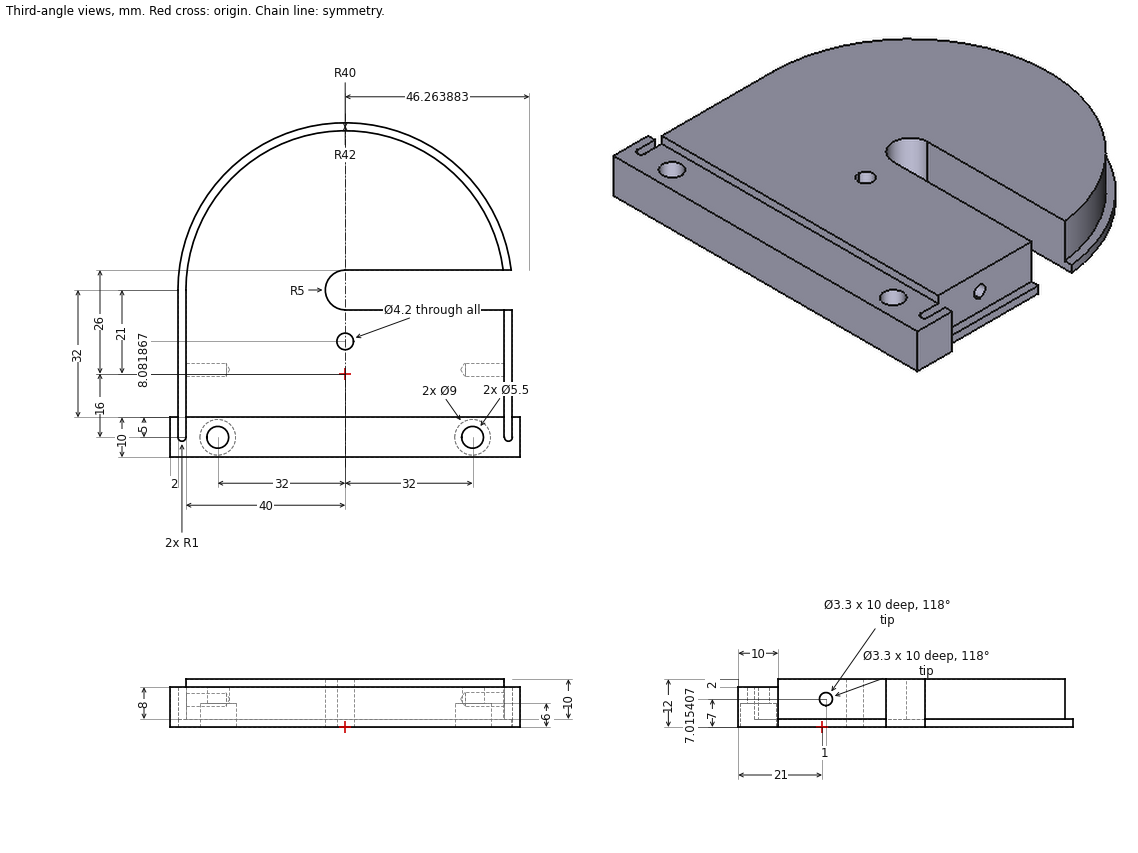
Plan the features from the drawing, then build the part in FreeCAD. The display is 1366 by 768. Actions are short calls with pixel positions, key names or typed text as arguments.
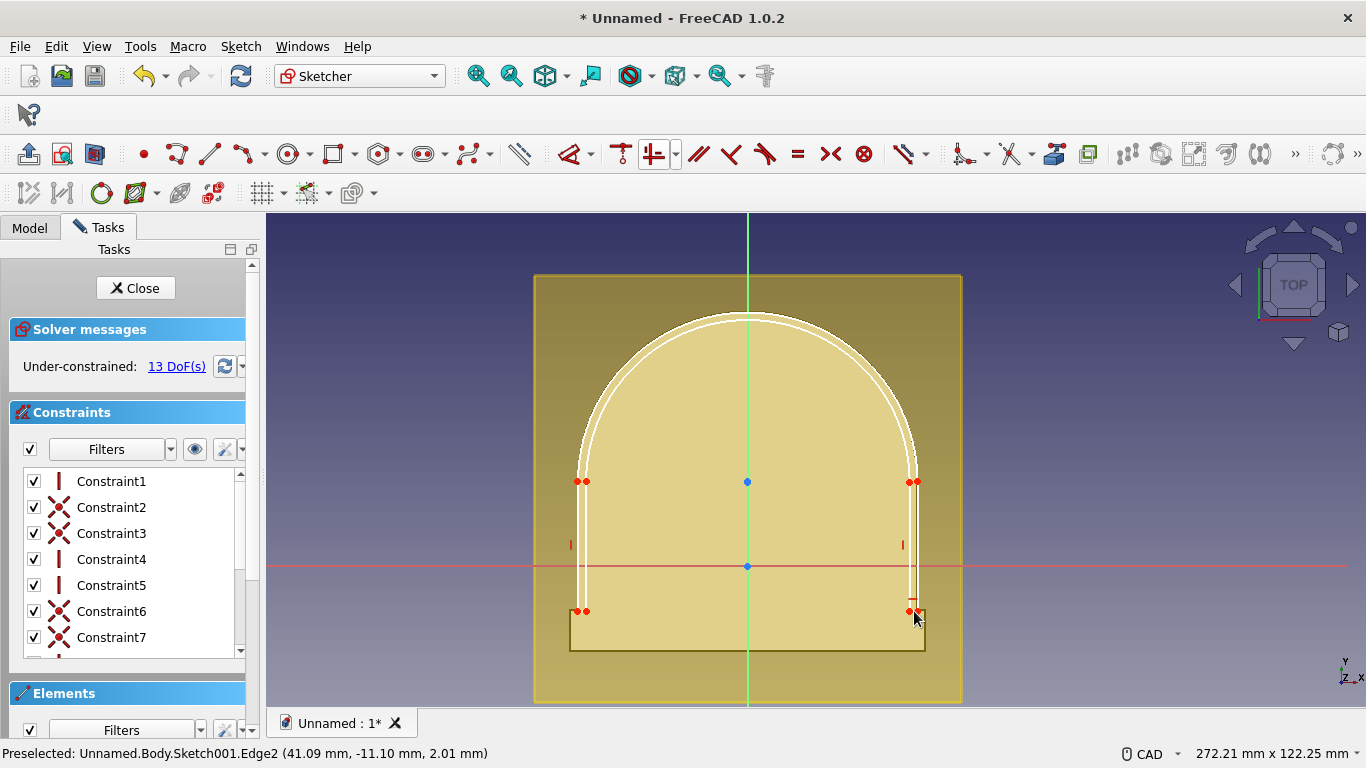
scroll(580, 612, up, 9)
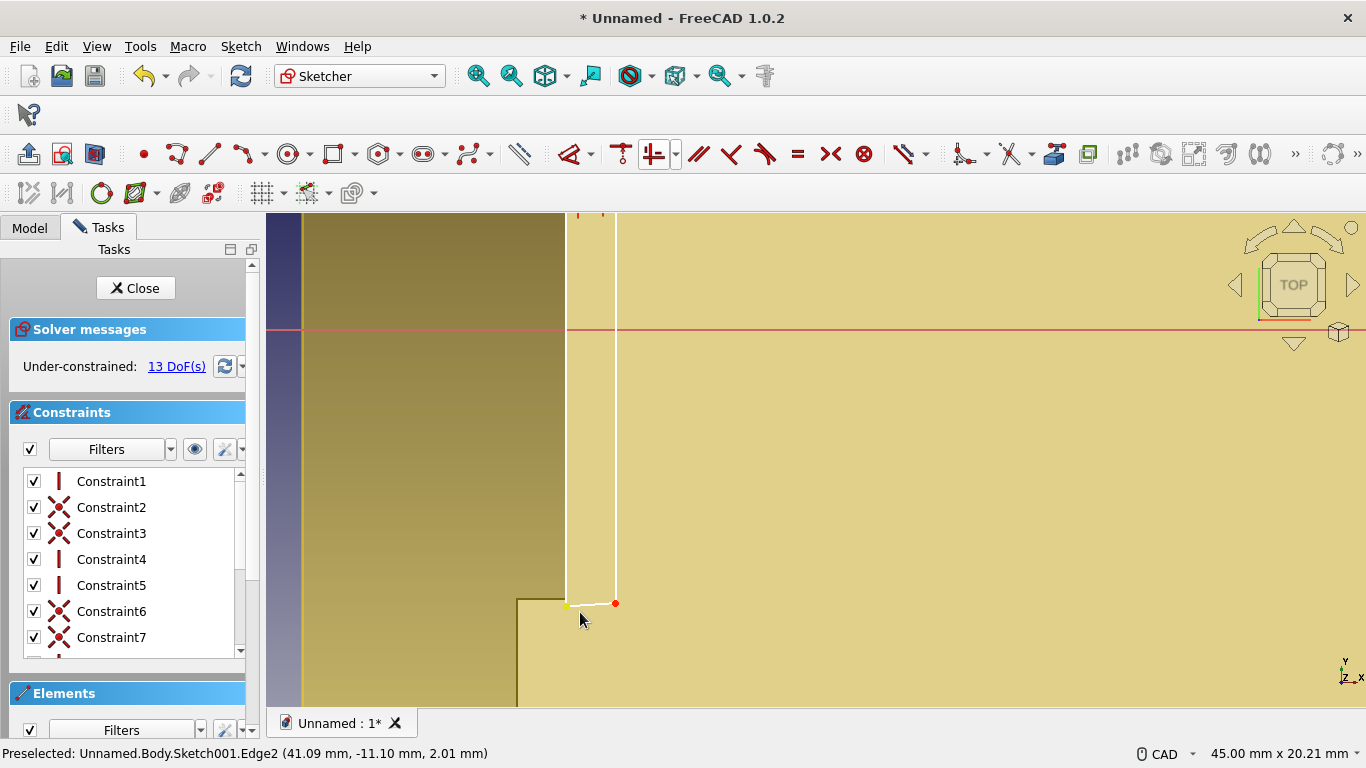
click(581, 605)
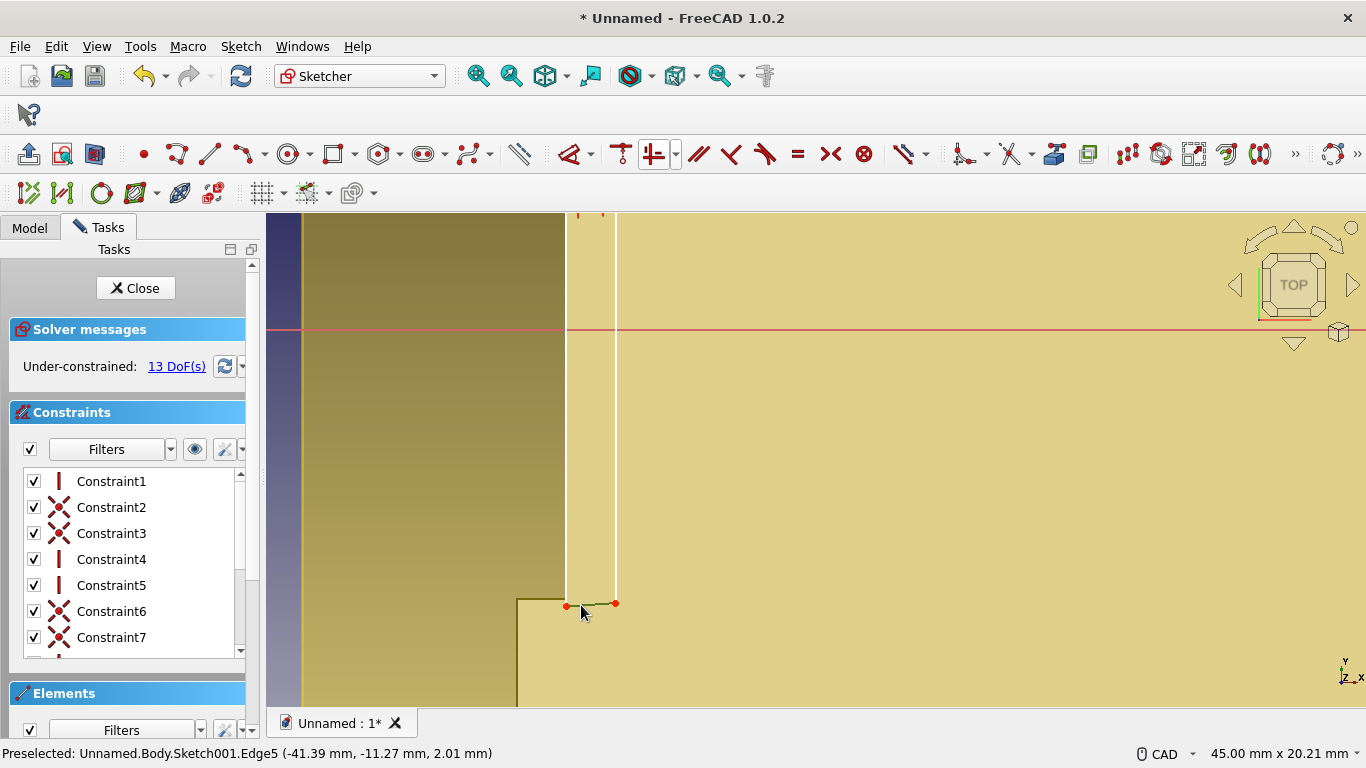
key(h)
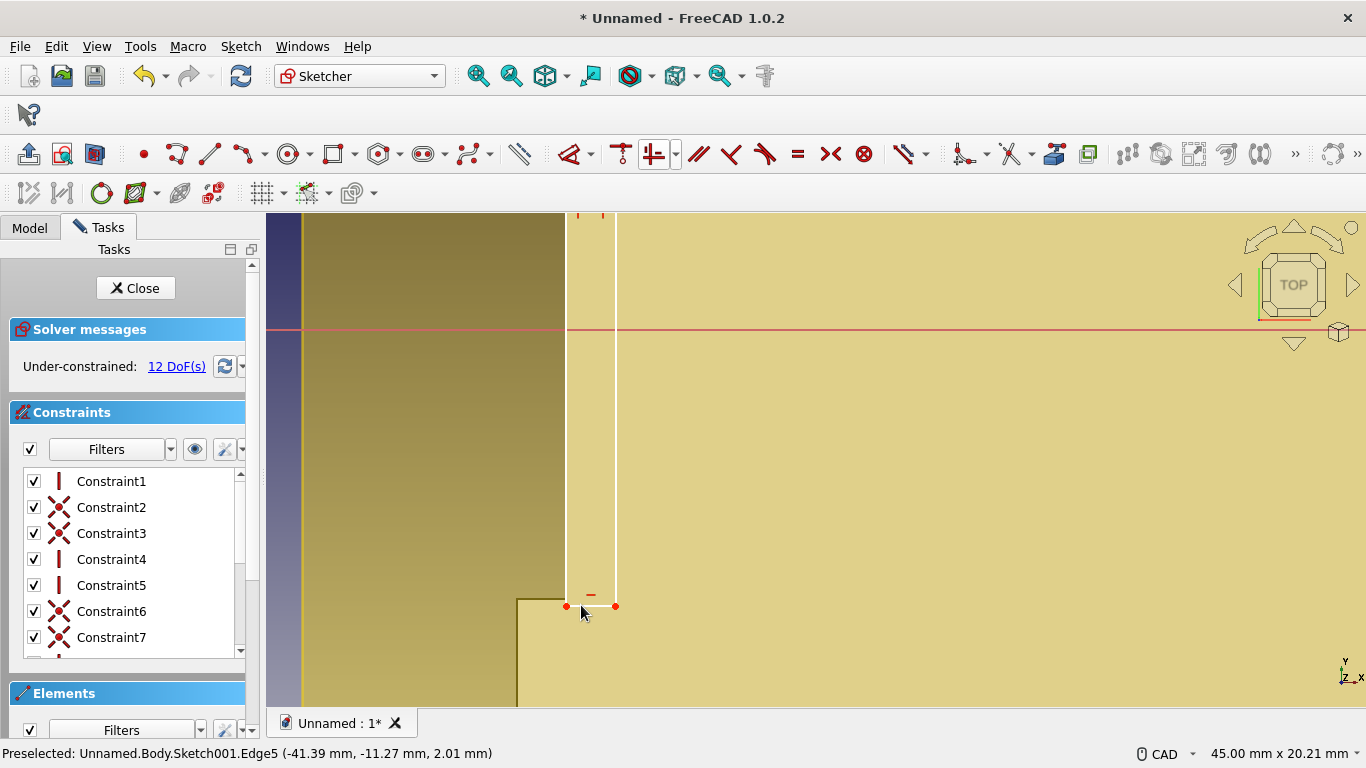
scroll(580, 612, down, 9)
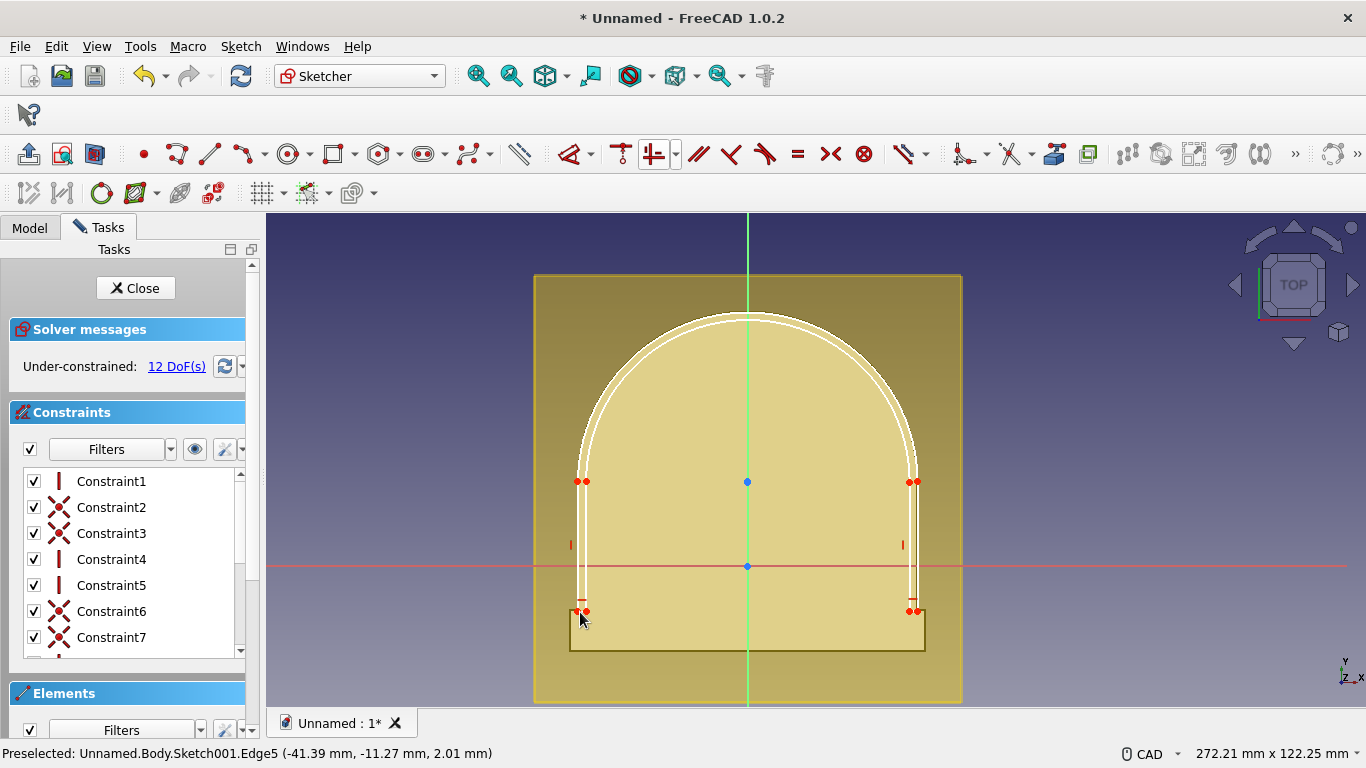
scroll(847, 345, up, 4)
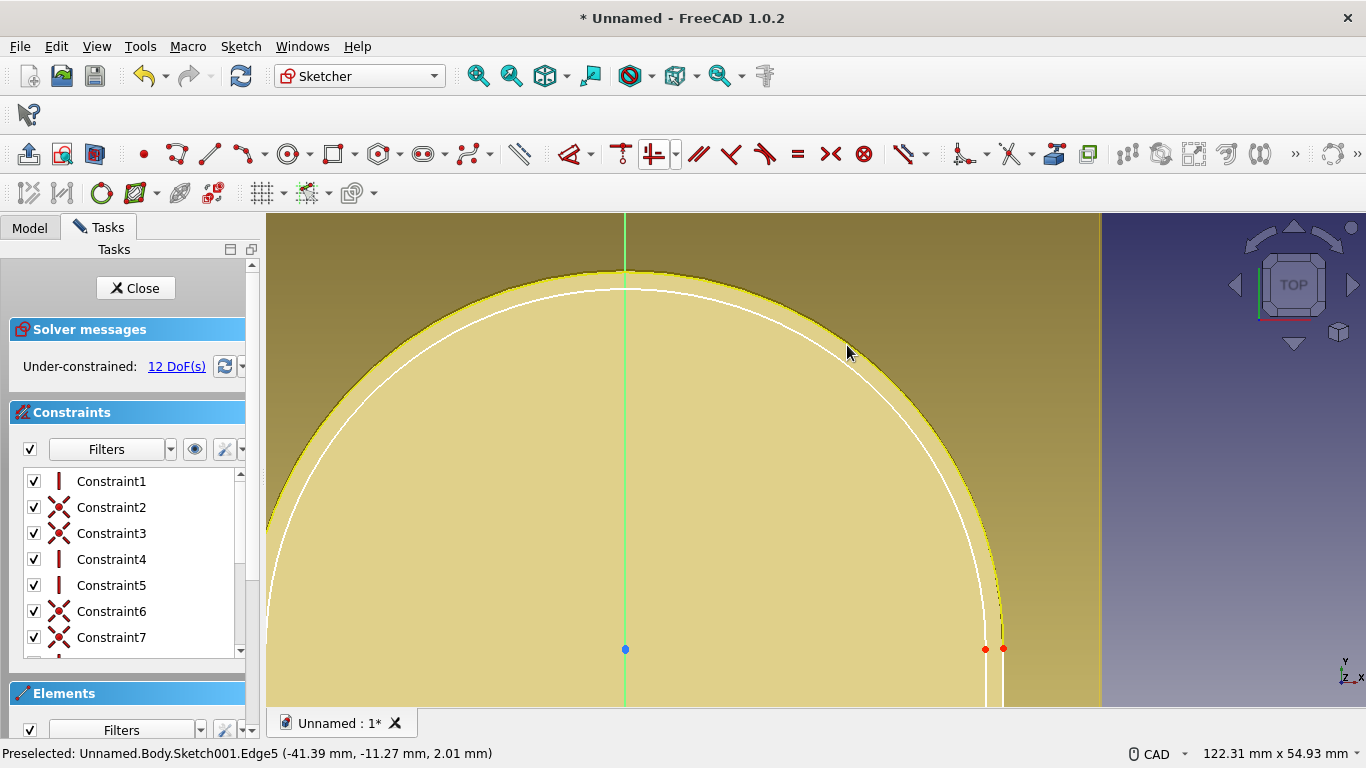
click(847, 344)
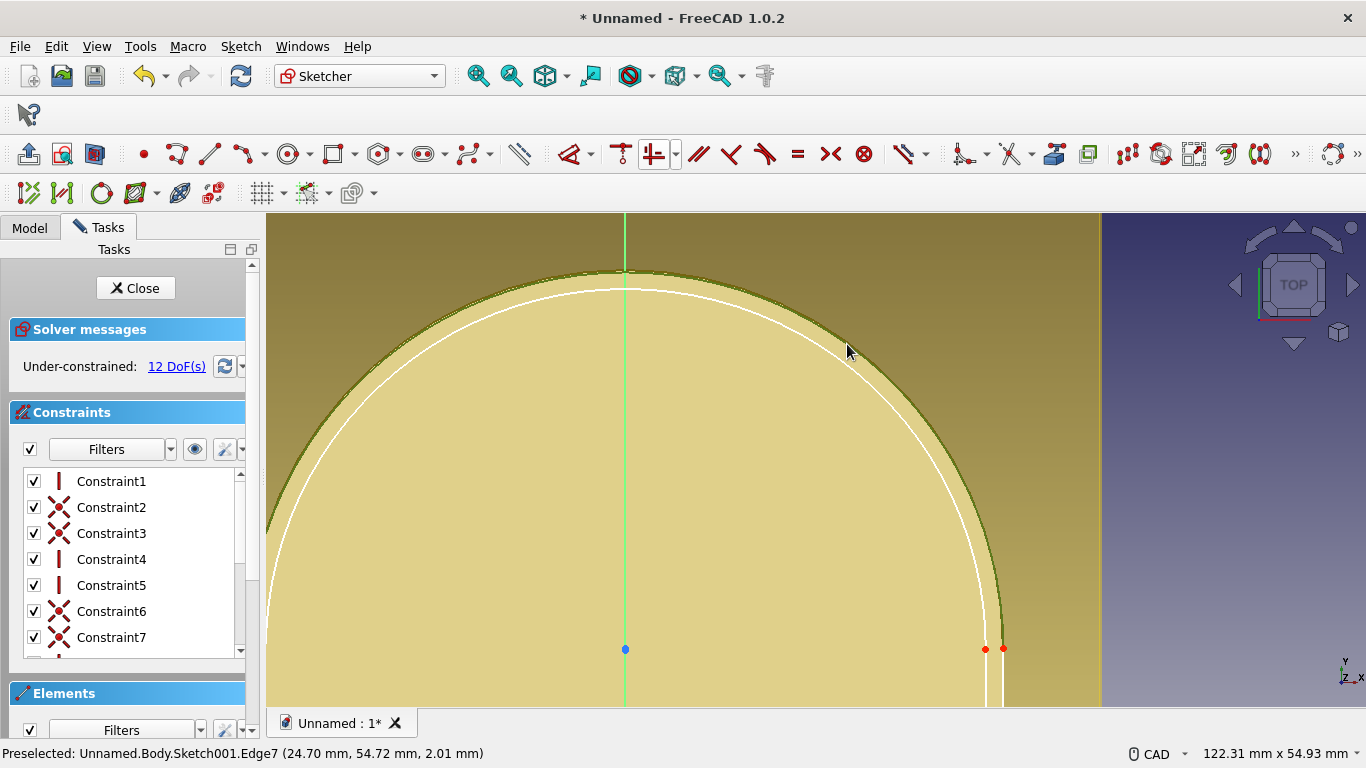
click(838, 358)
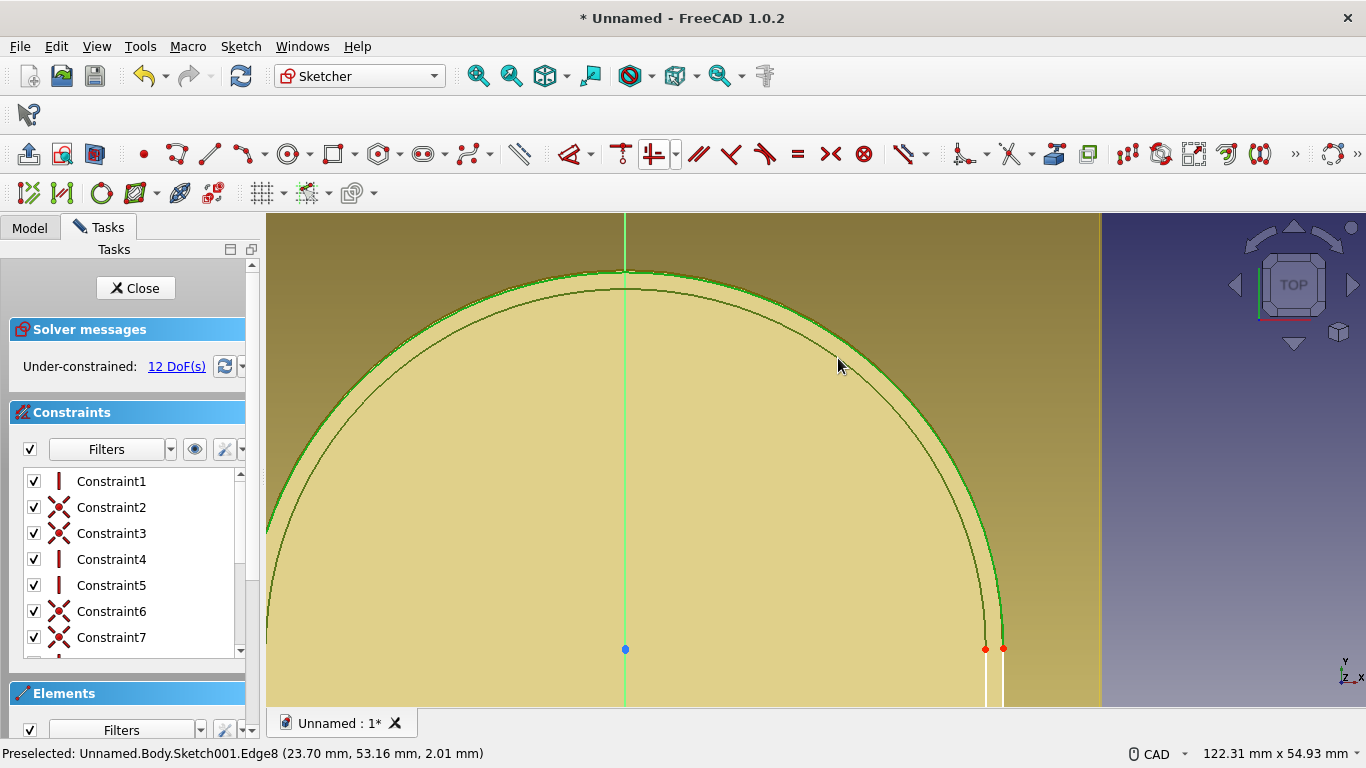
key(c)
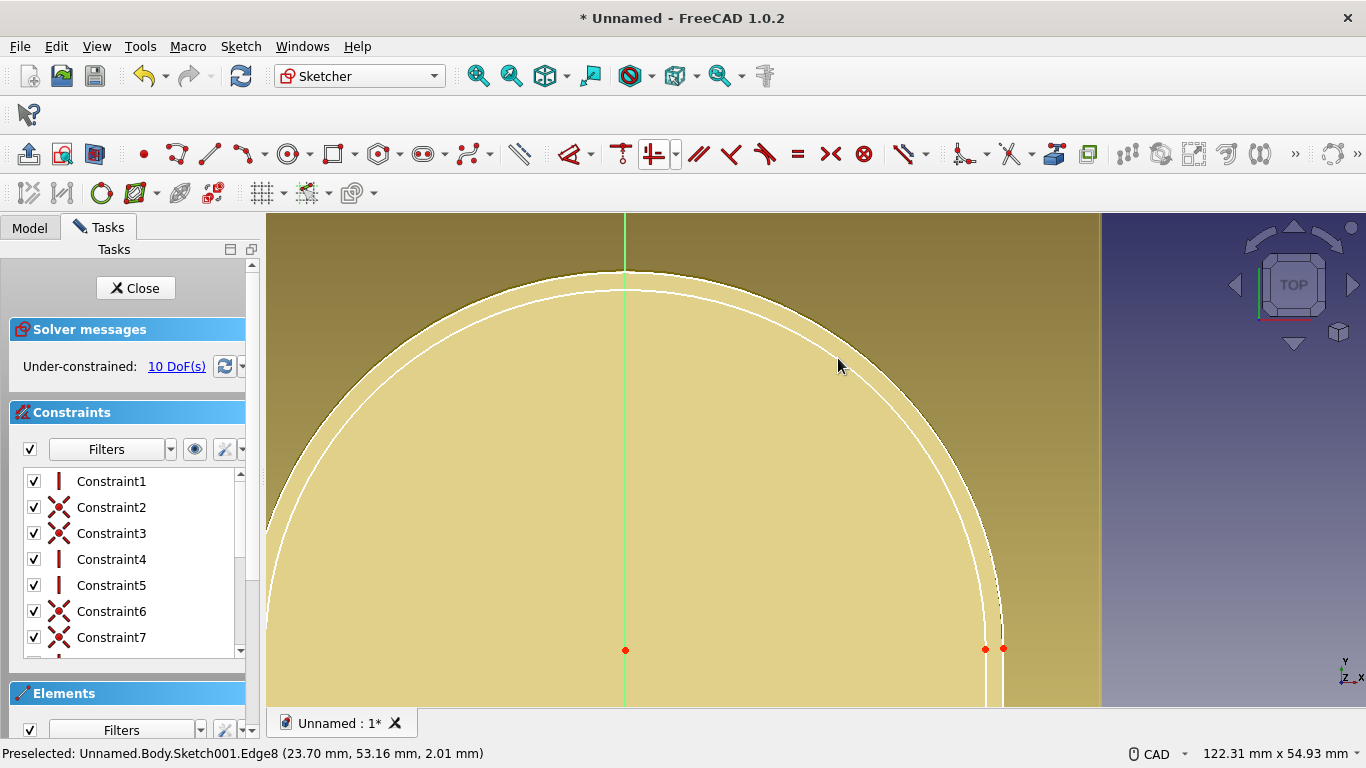
click(626, 650)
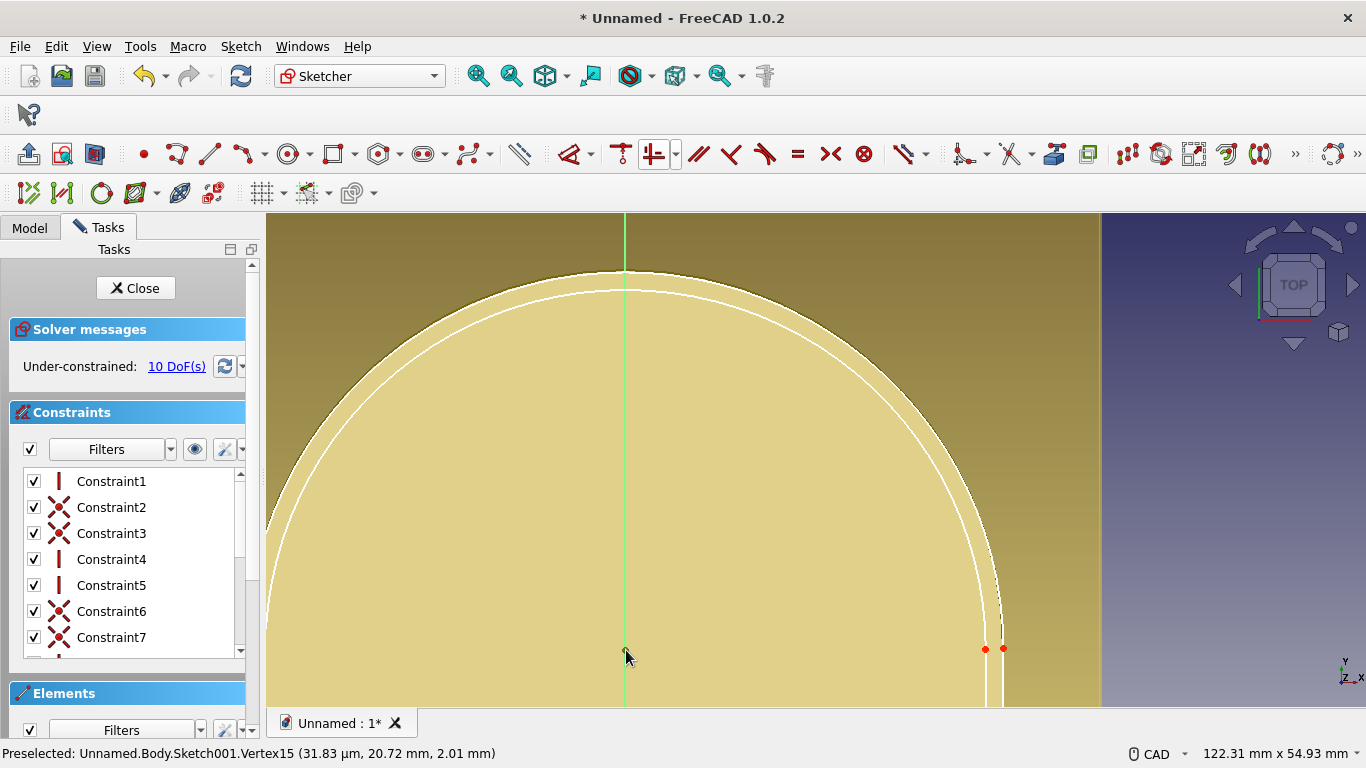
click(625, 616)